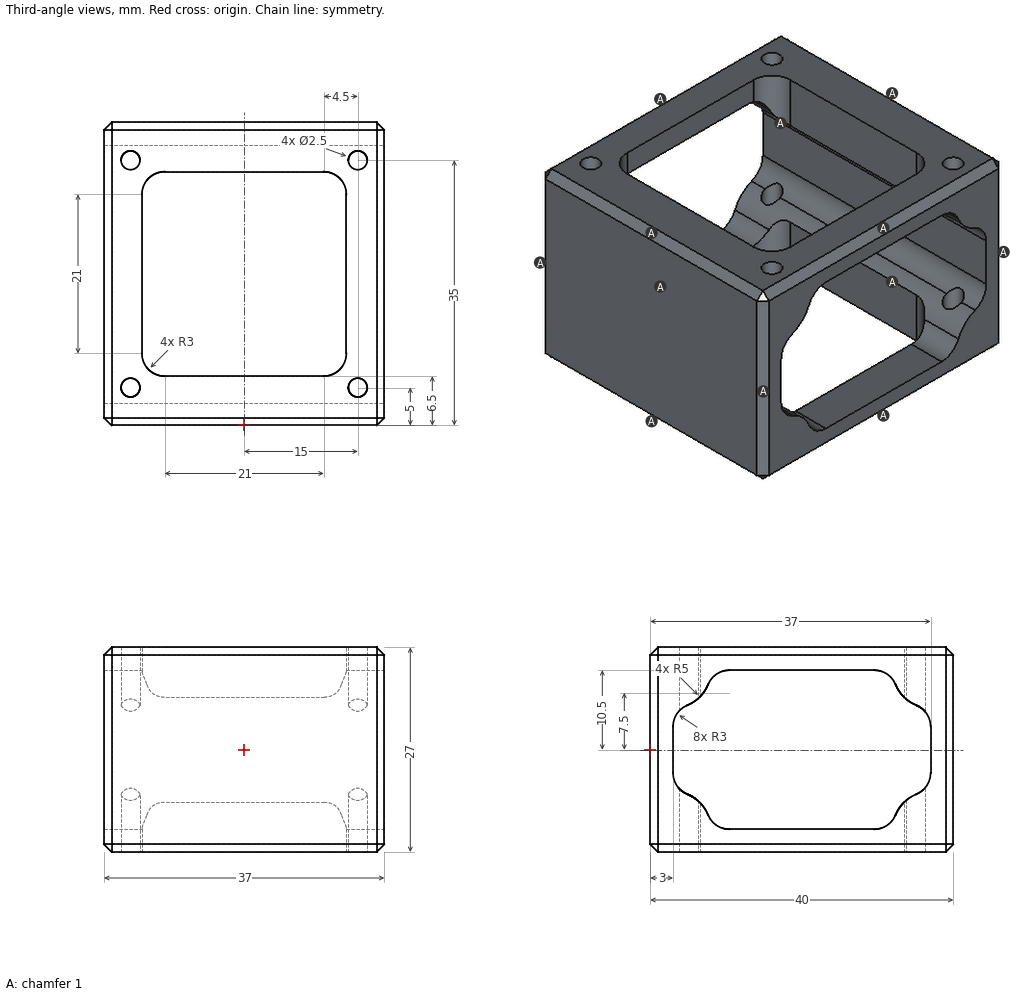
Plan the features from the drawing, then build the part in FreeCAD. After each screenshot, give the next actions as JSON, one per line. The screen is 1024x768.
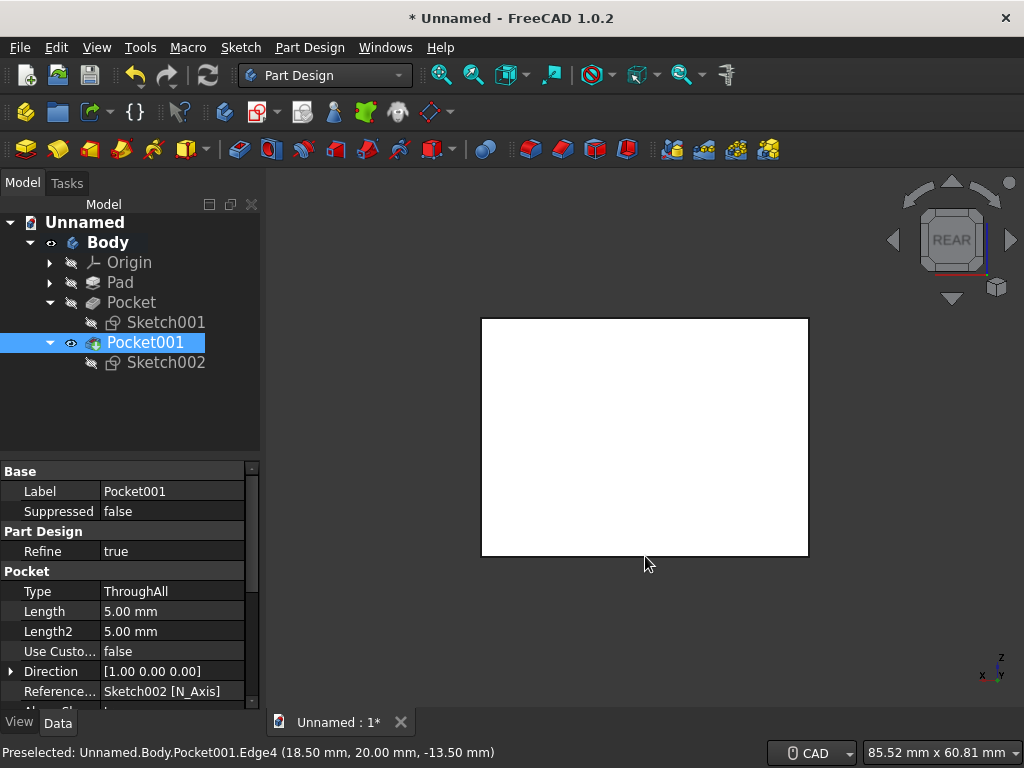
{"action": "left_click", "coordinate": [645, 437], "text": "ctrl"}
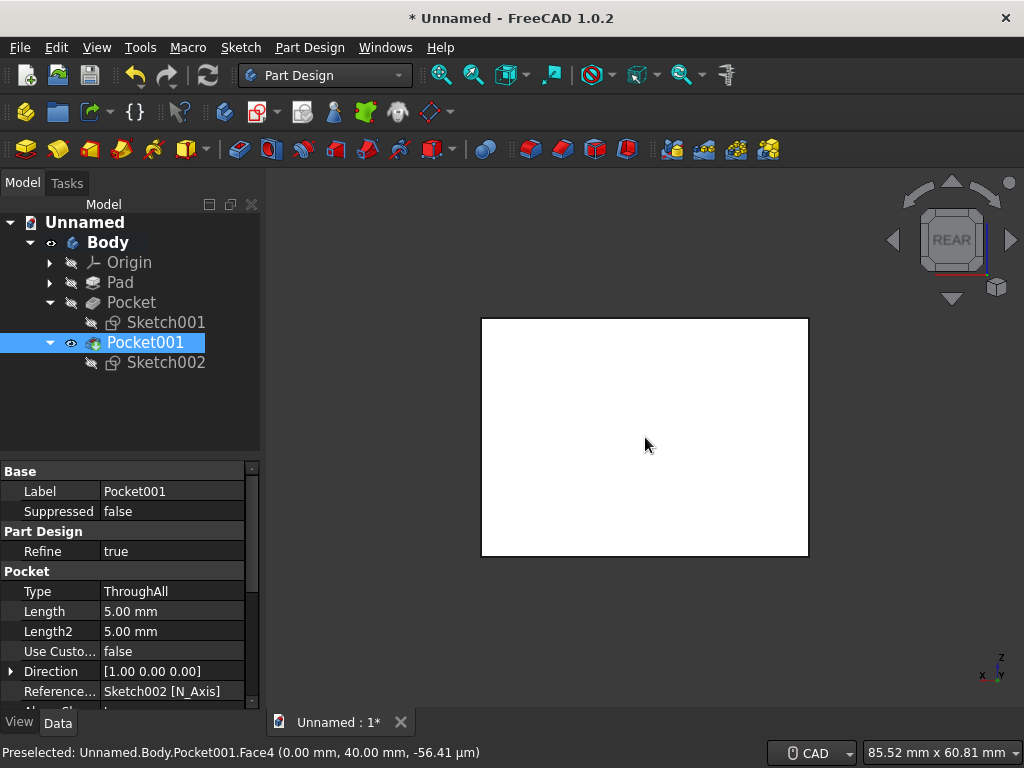
{"action": "left_click", "coordinate": [564, 150]}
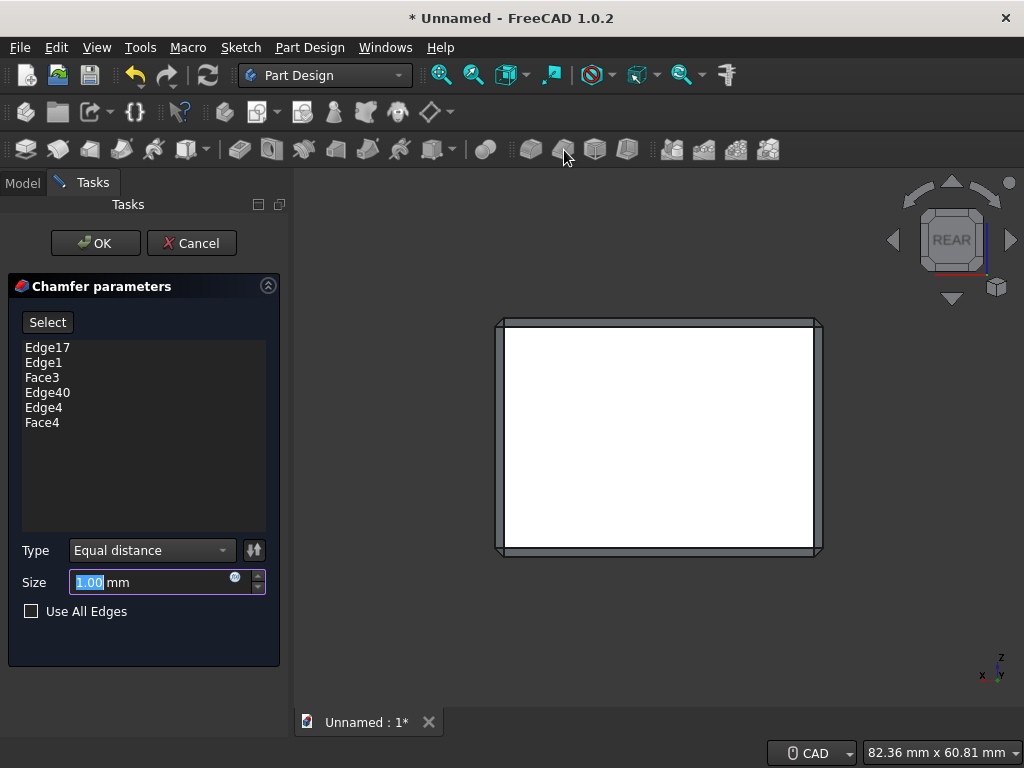
{"action": "type", "text": "1"}
{"action": "key", "text": "Tab"}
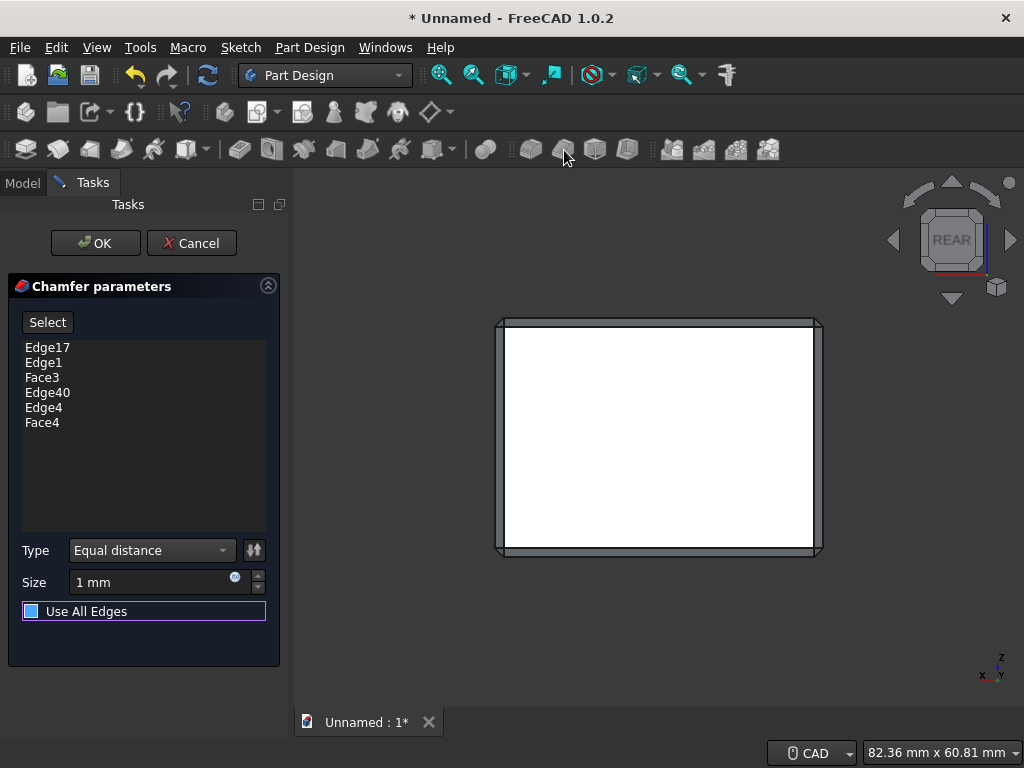
{"action": "left_click", "coordinate": [96, 243]}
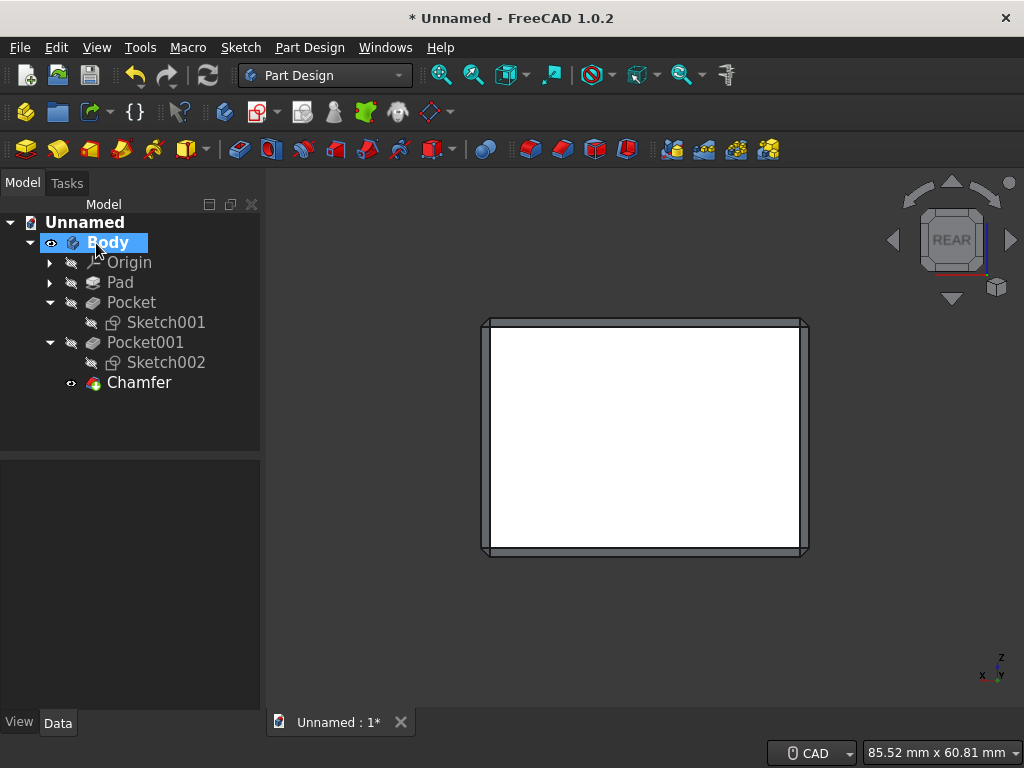
{"action": "key", "text": "0"}